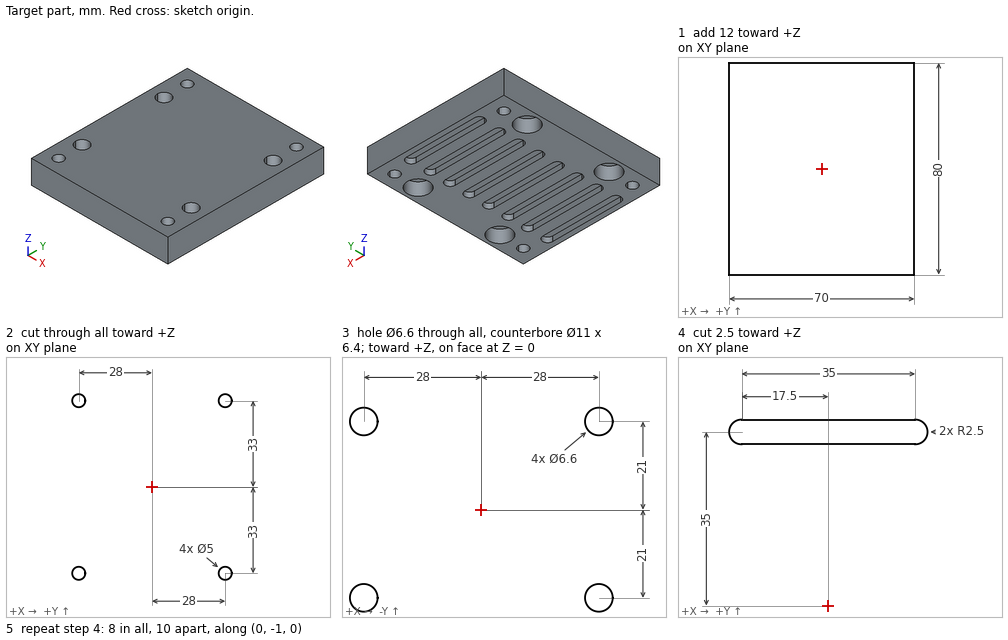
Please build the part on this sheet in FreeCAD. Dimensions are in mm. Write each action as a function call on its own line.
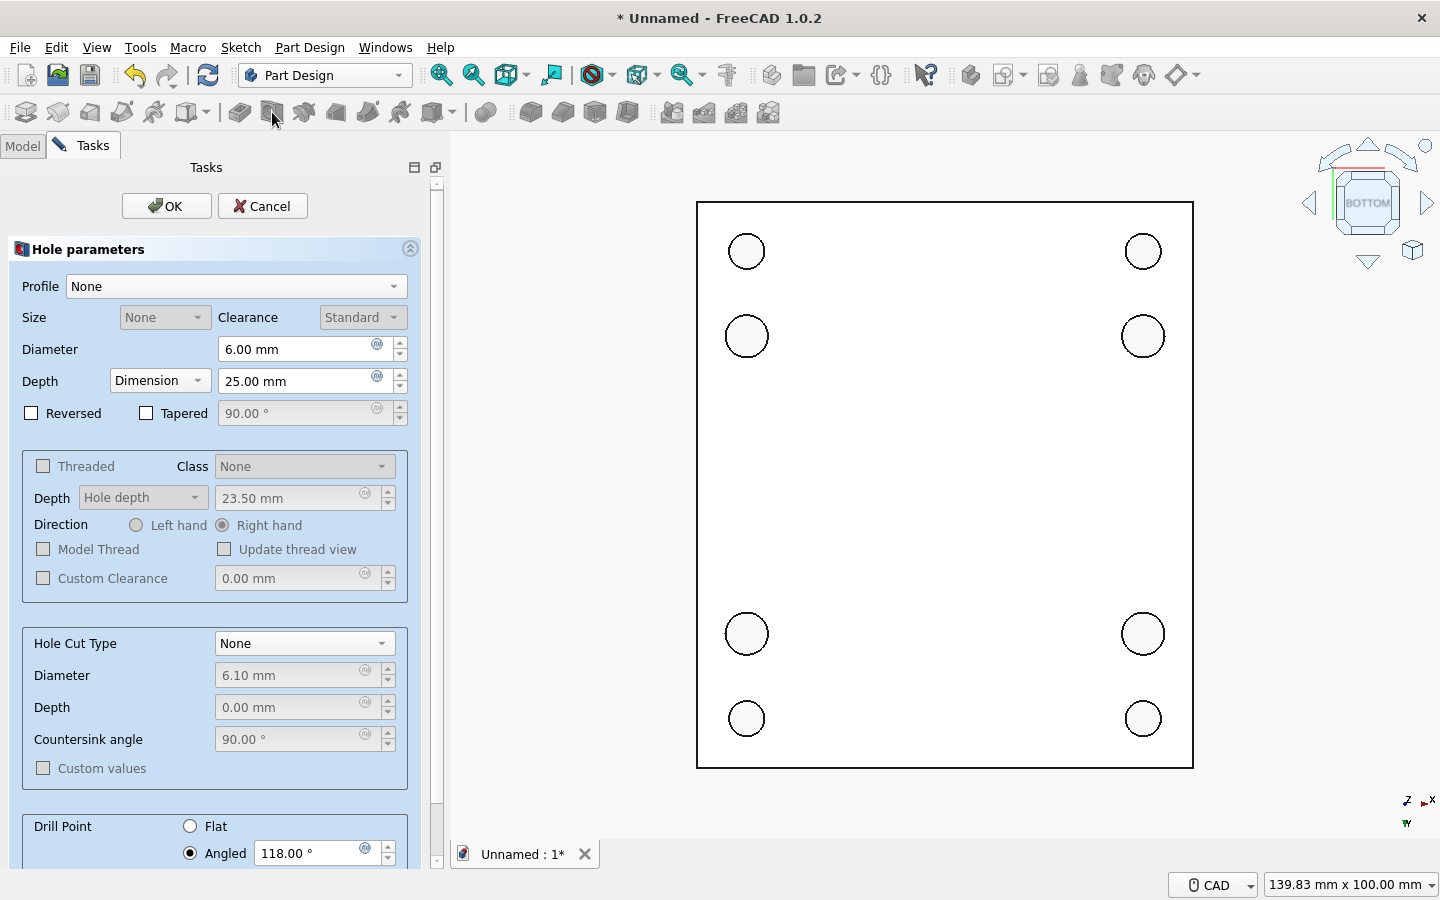
triple_click(305, 349)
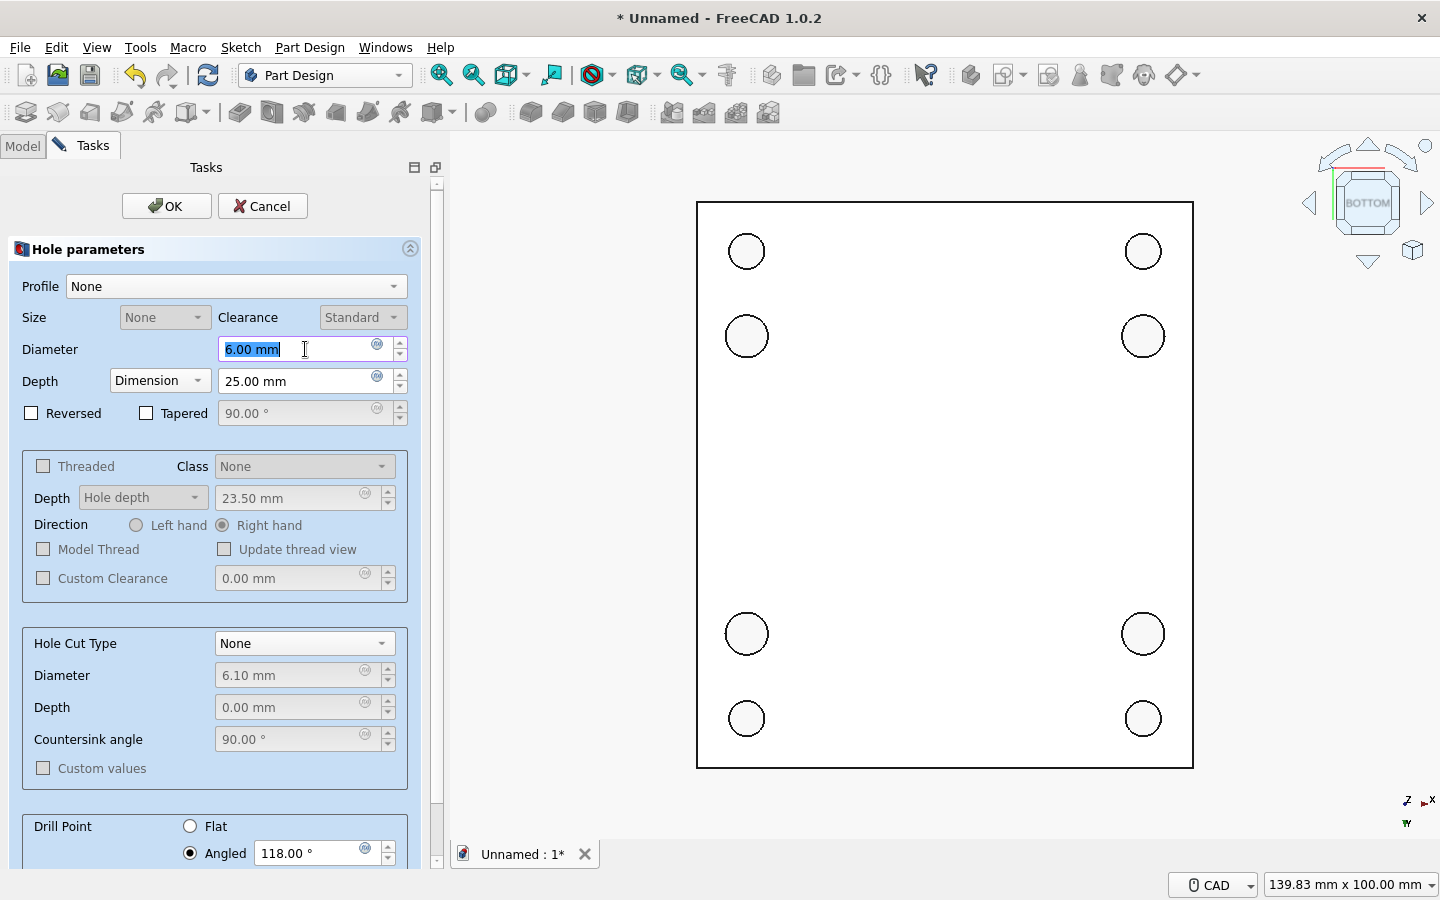
text(6.6)
key(Tab)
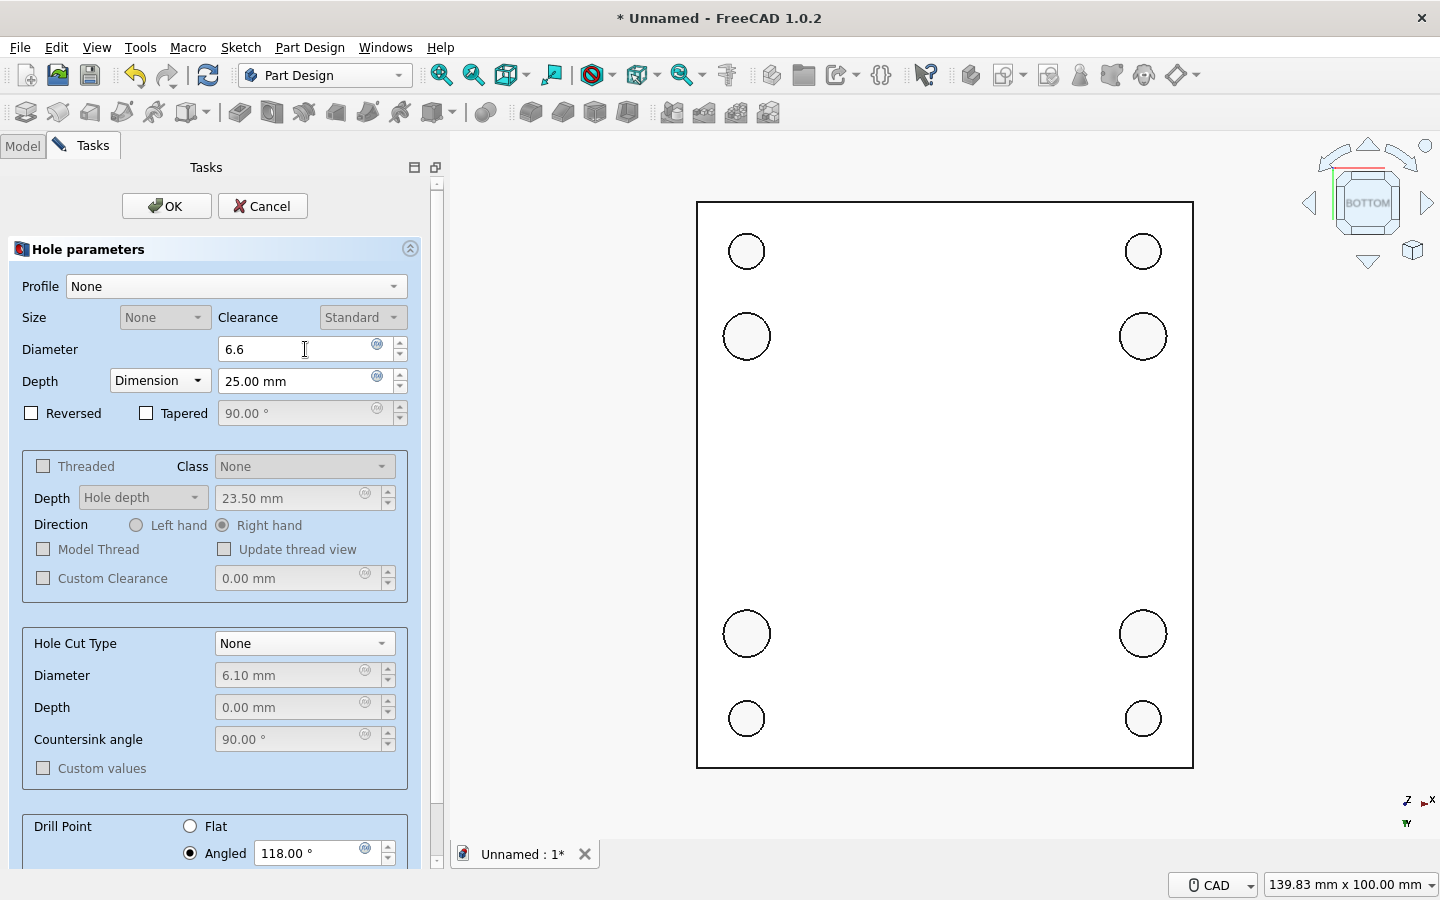
click(161, 380)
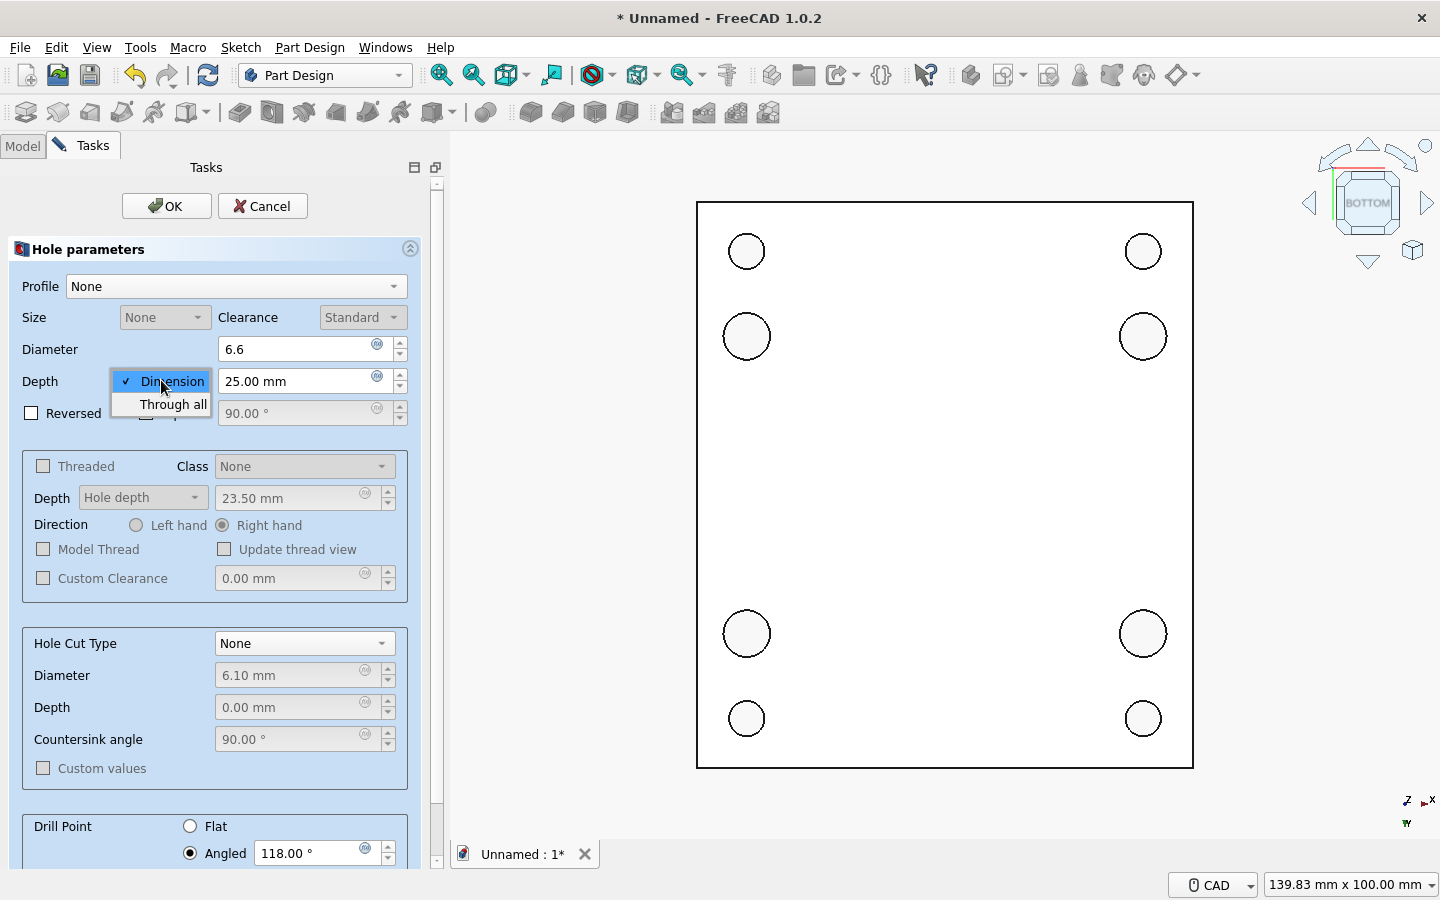
click(160, 404)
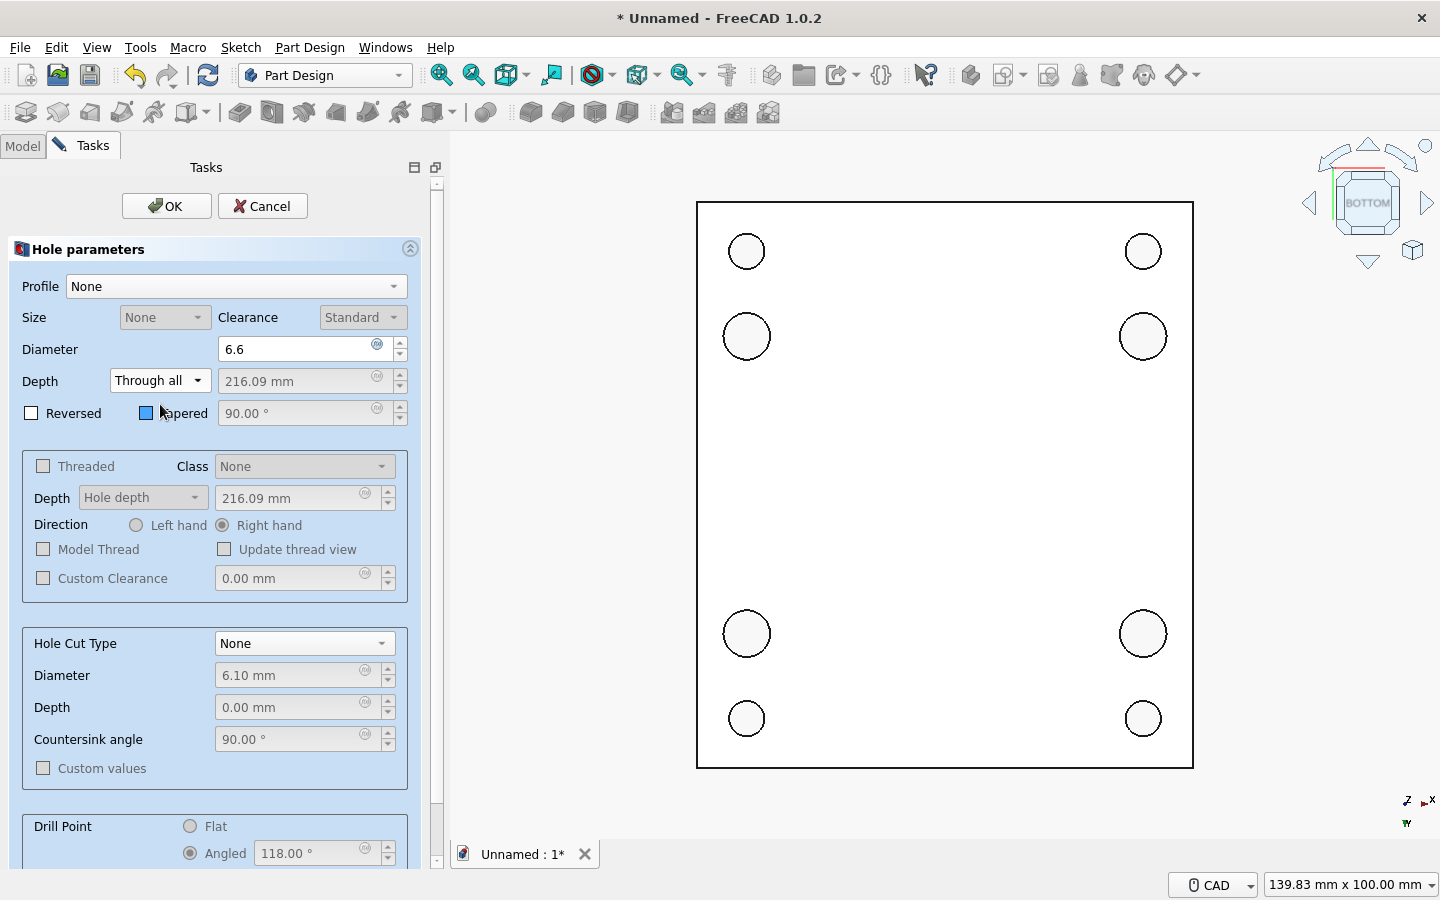
click(306, 644)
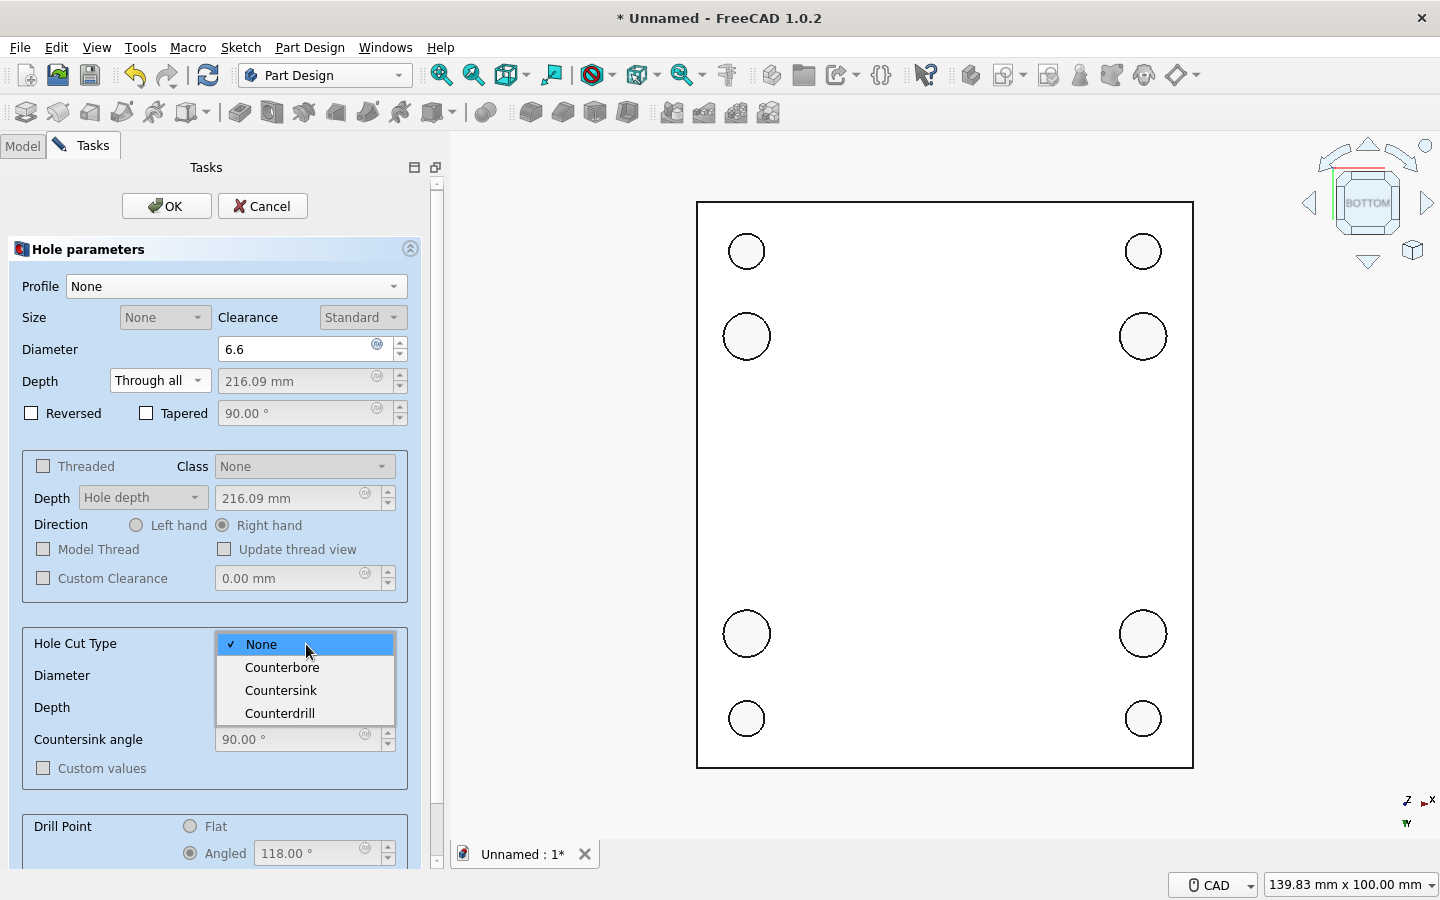
click(304, 668)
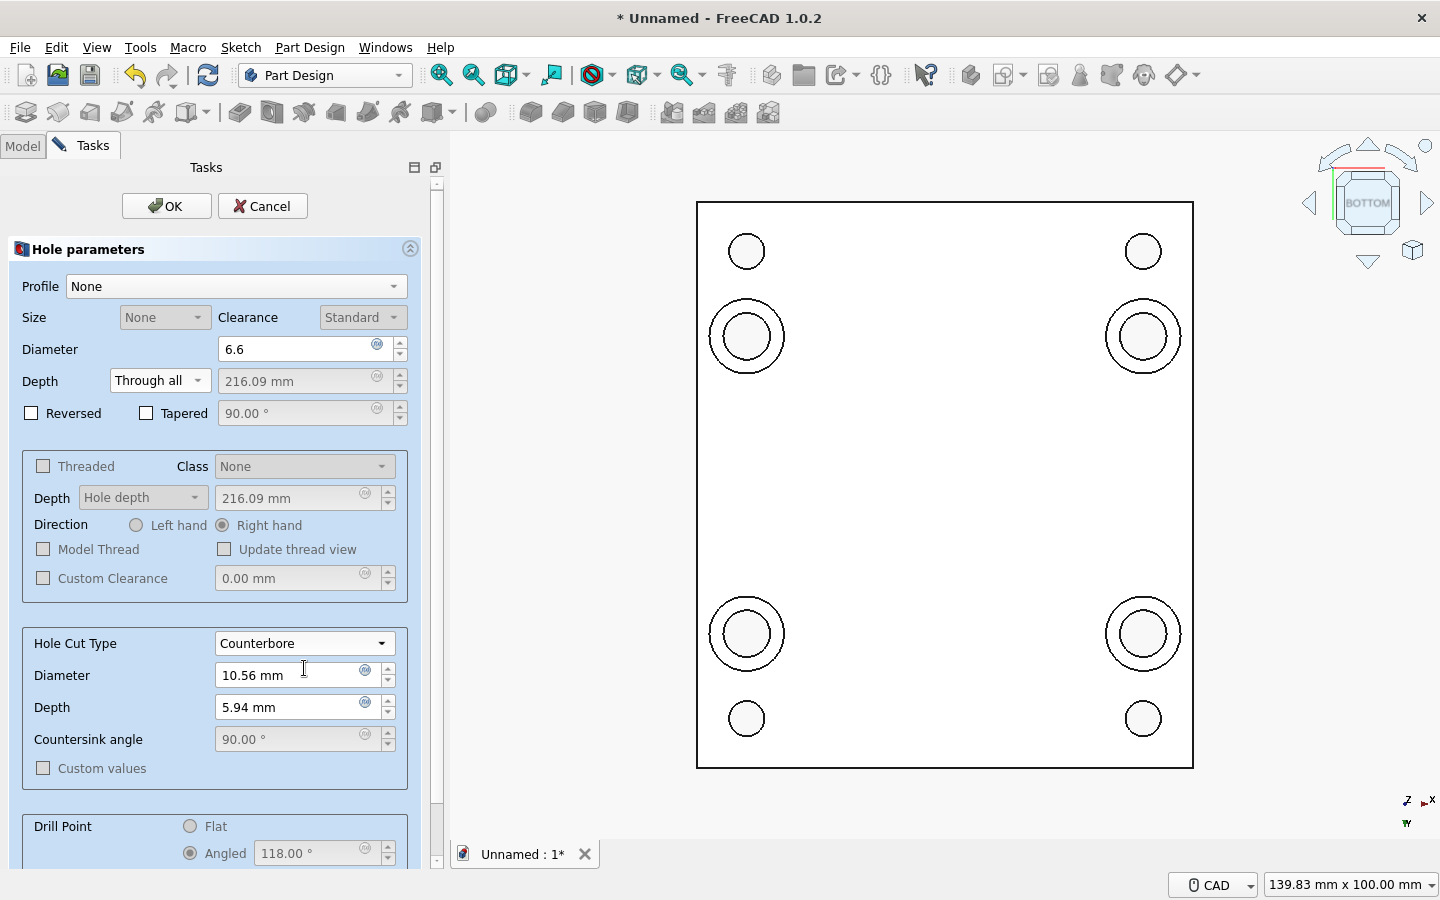
triple_click(298, 675)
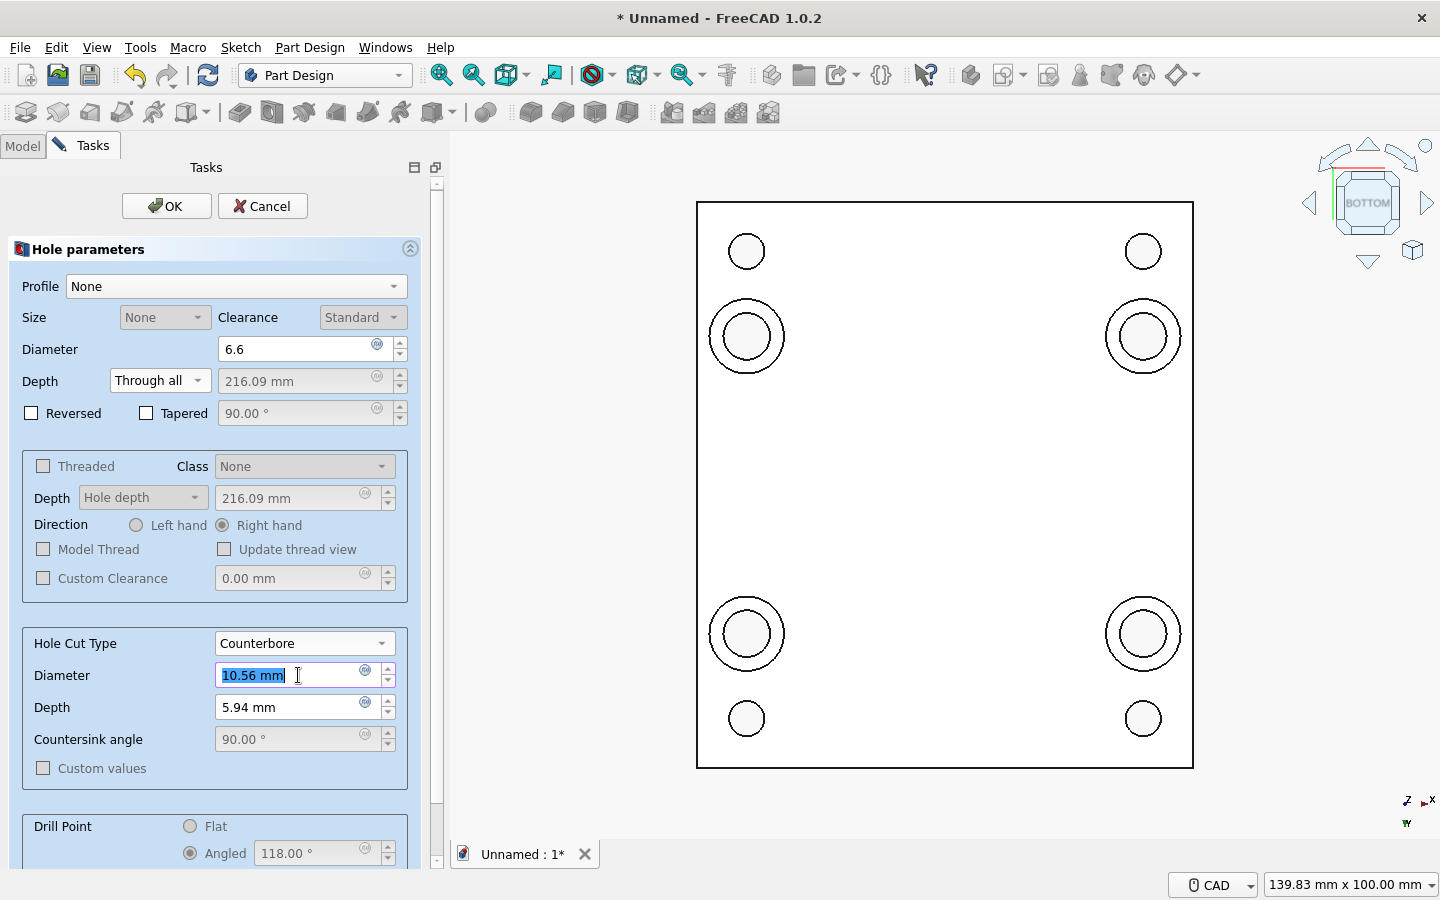
text(11)
key(Tab)